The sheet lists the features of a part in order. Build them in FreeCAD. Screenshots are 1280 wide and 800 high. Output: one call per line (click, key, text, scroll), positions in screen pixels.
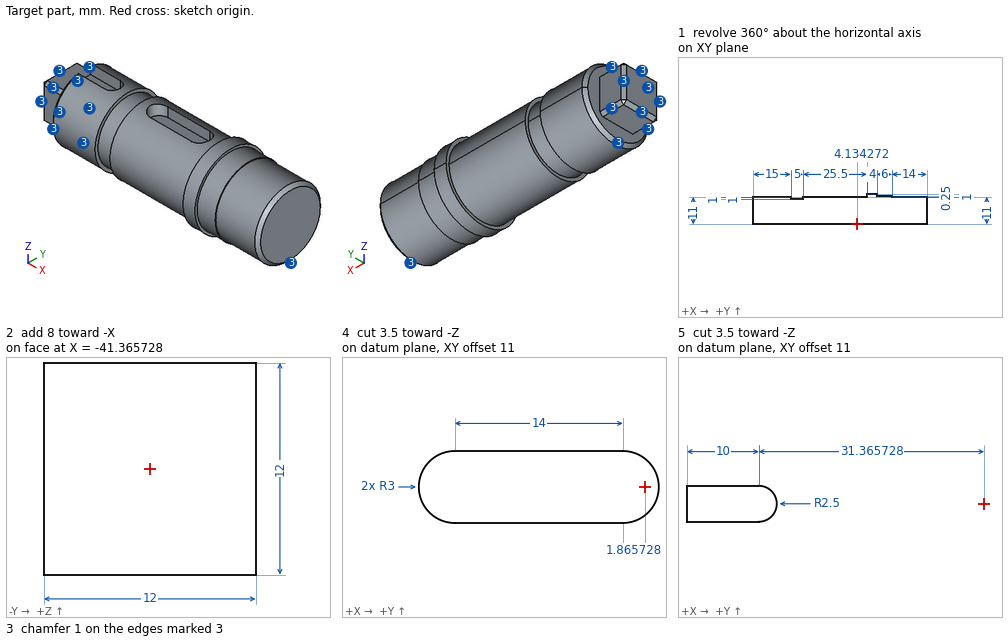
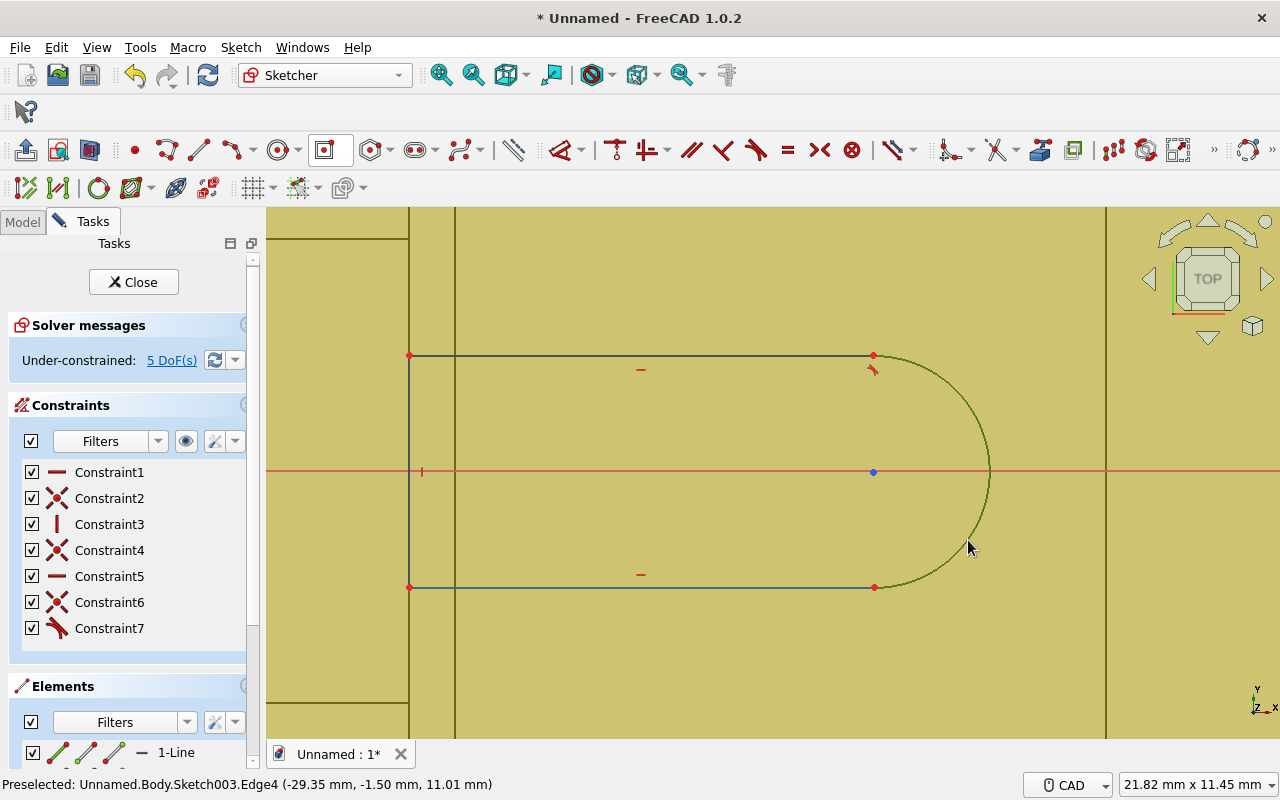
click(756, 150)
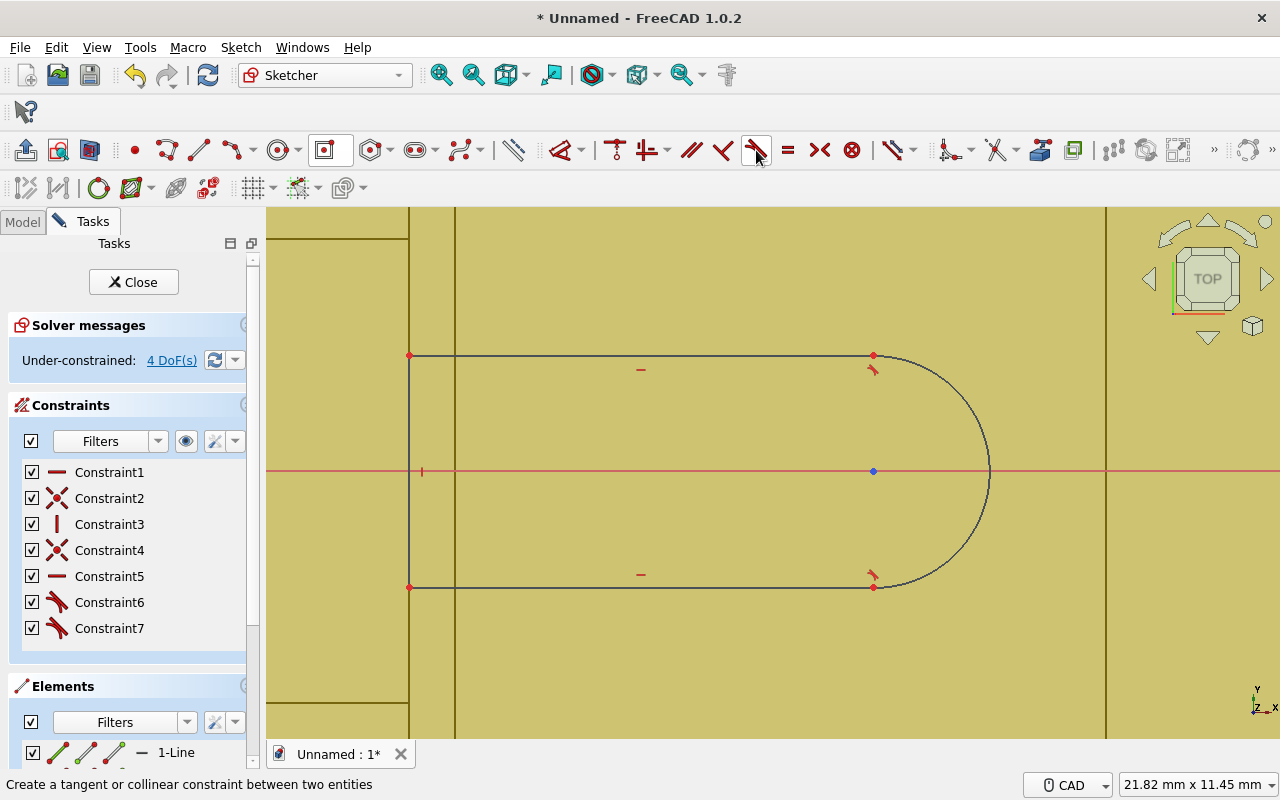
click(874, 472)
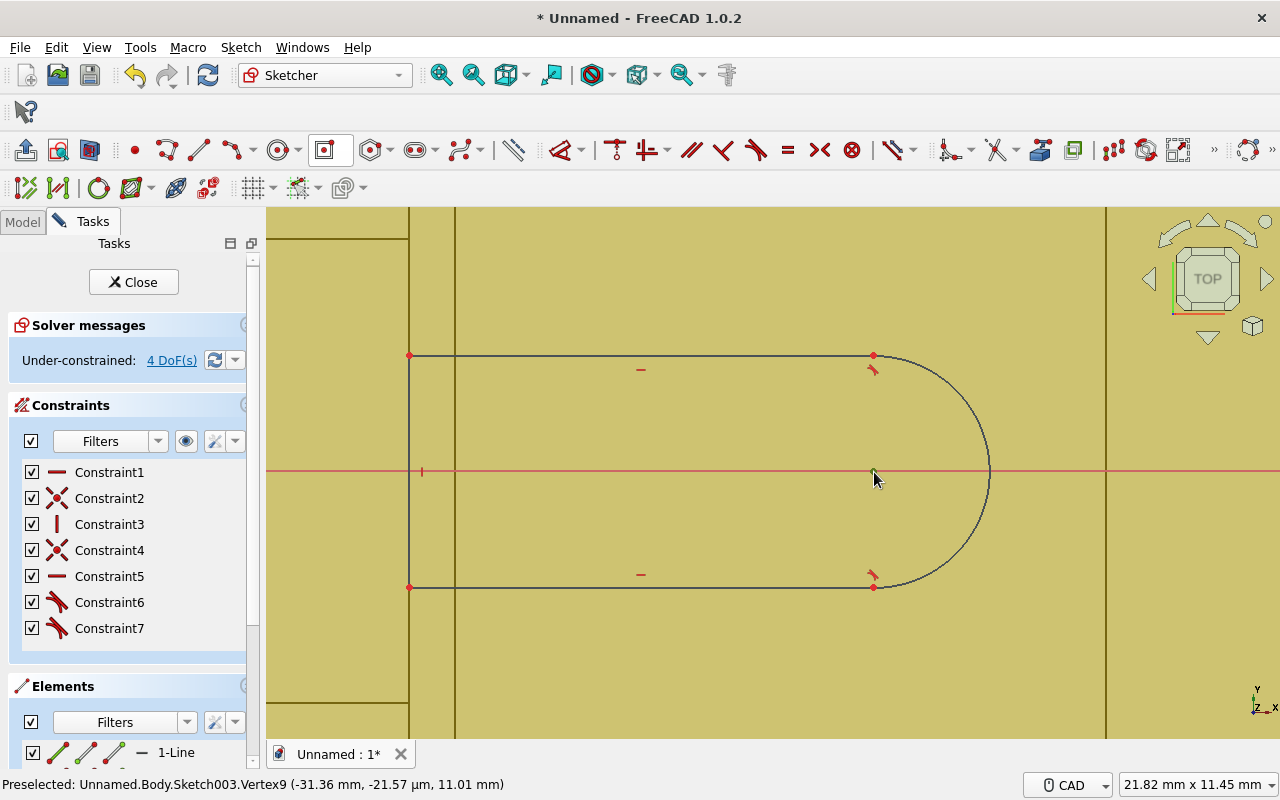
click(353, 471)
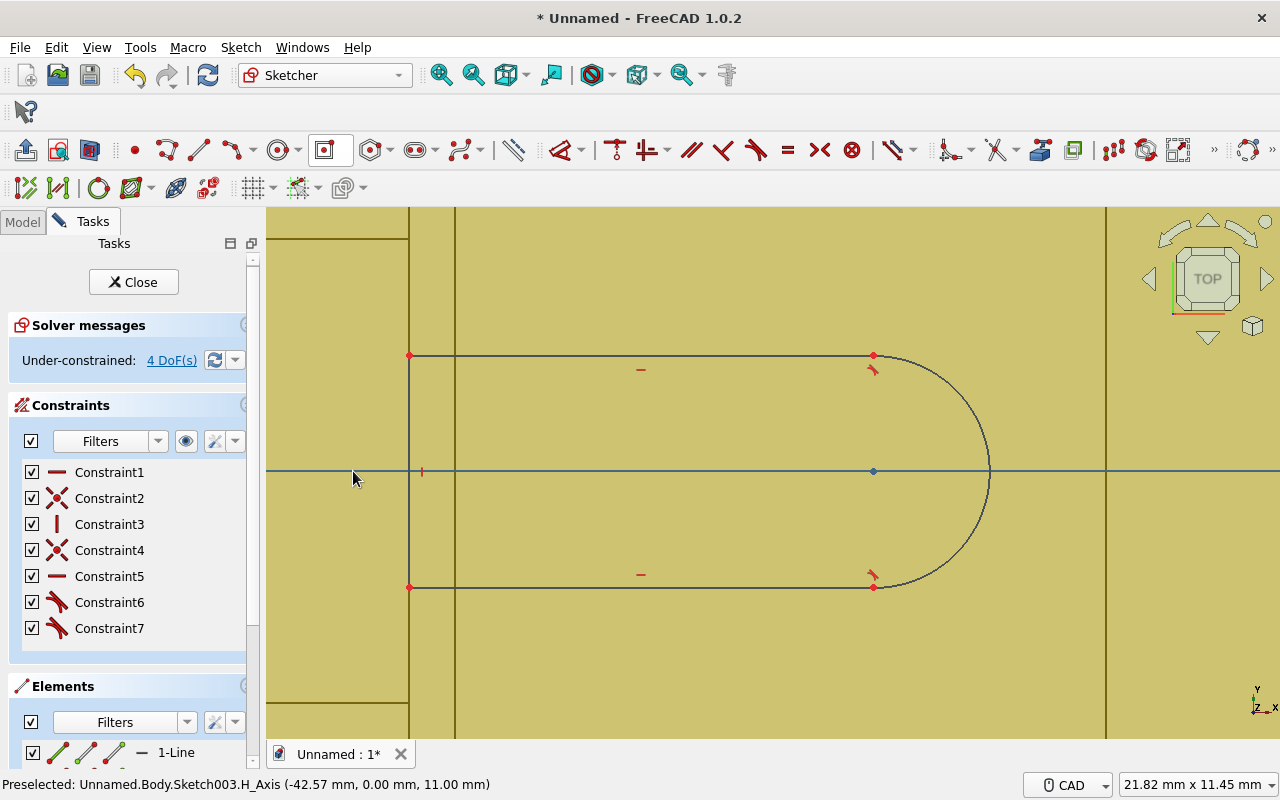
click(616, 150)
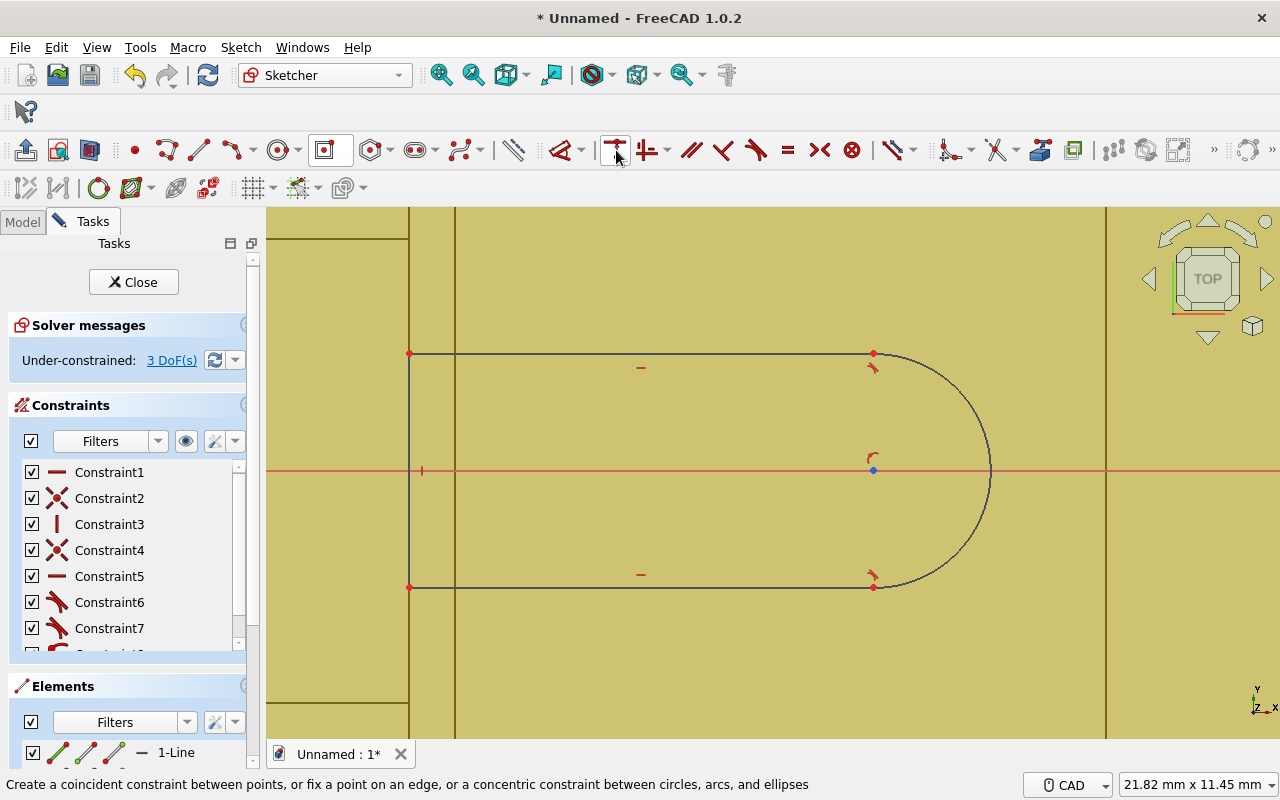
click(560, 150)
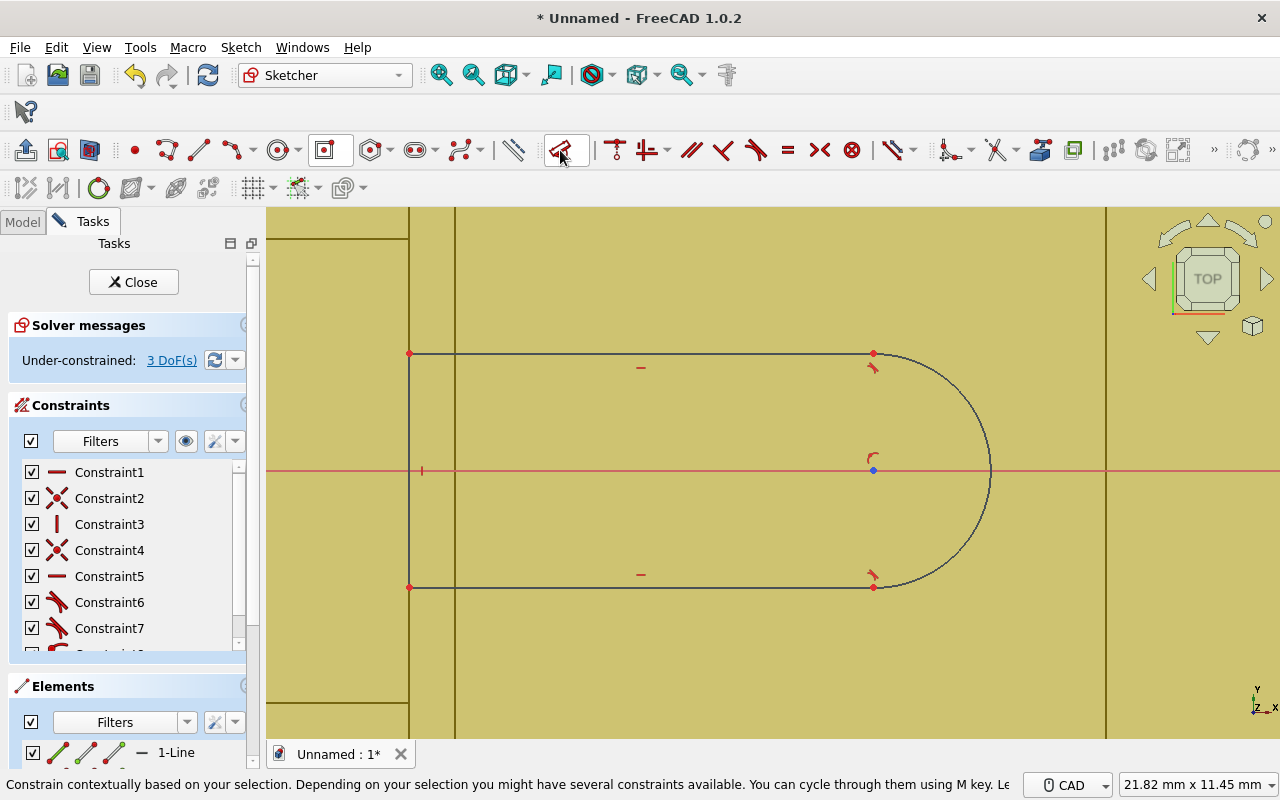
click(968, 540)
click(994, 559)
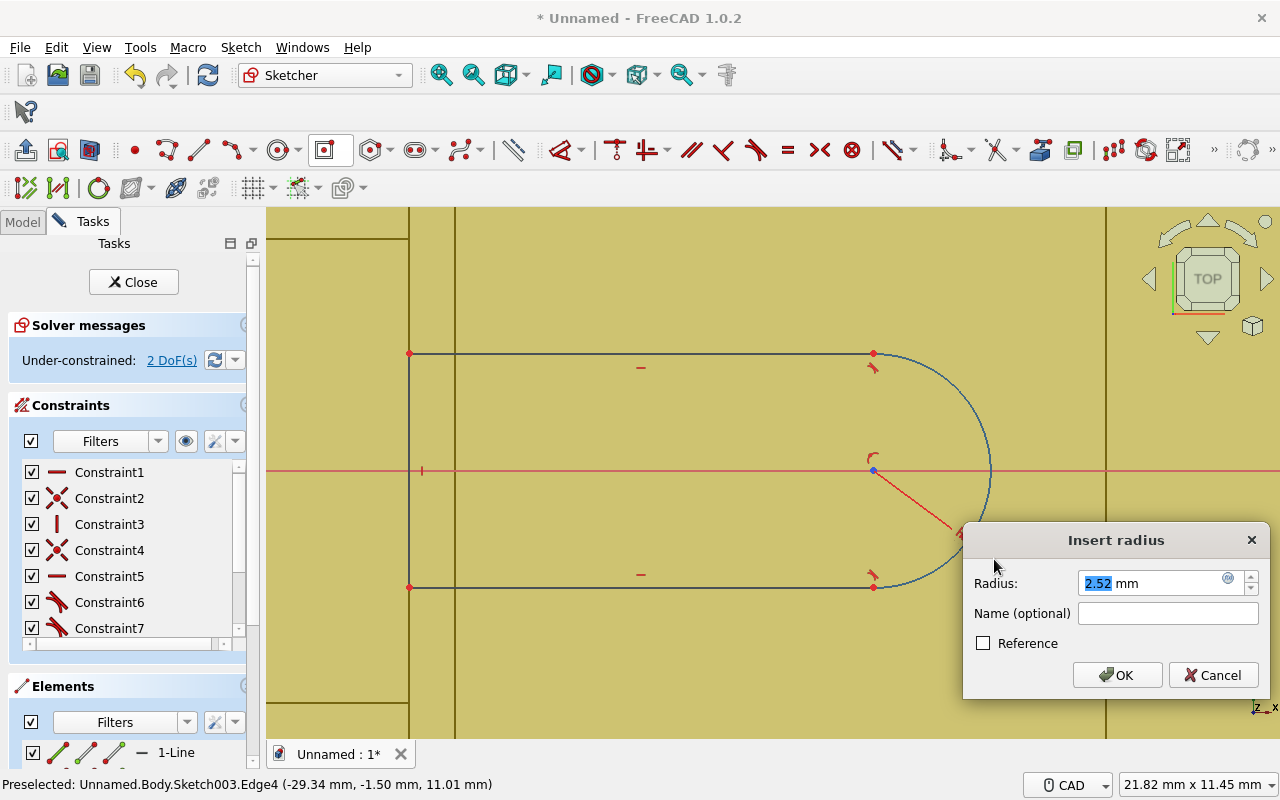
text(2.5)
key(Return)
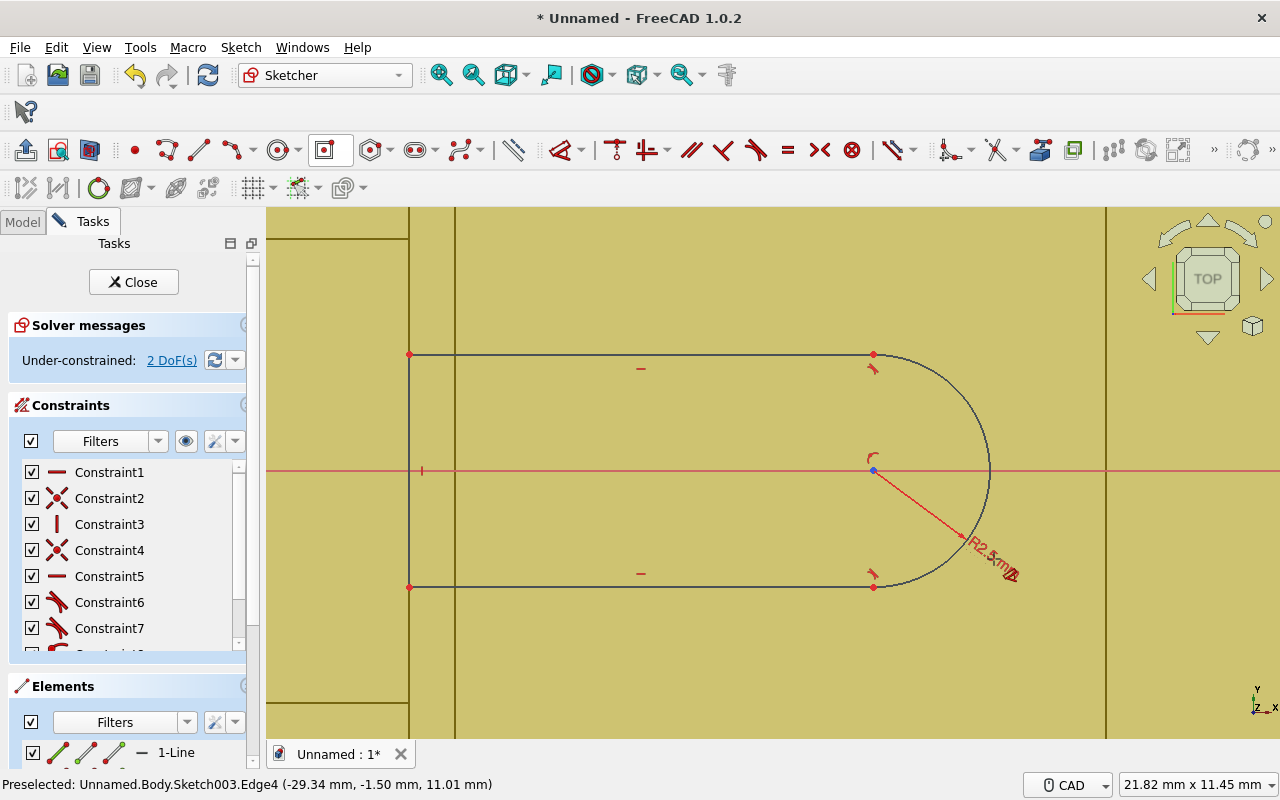
click(734, 355)
click(641, 321)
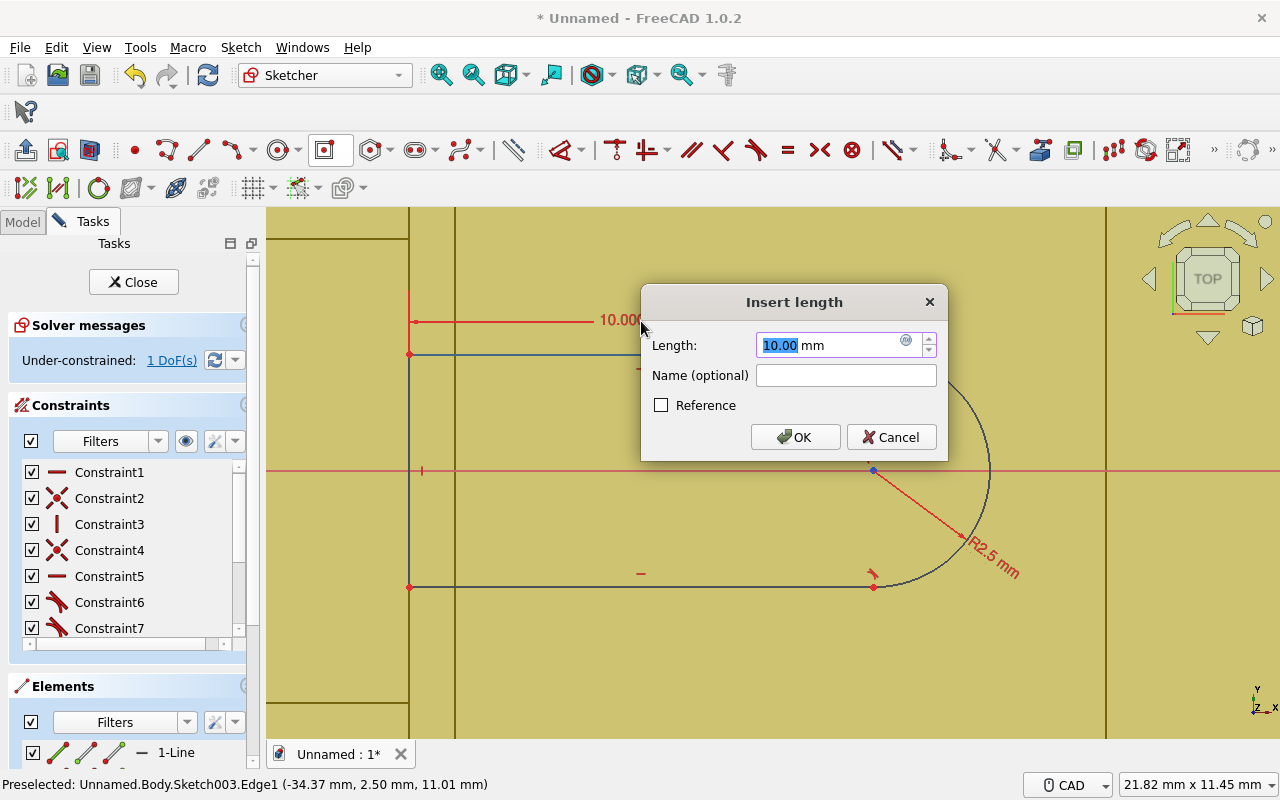
text(10)
key(Return)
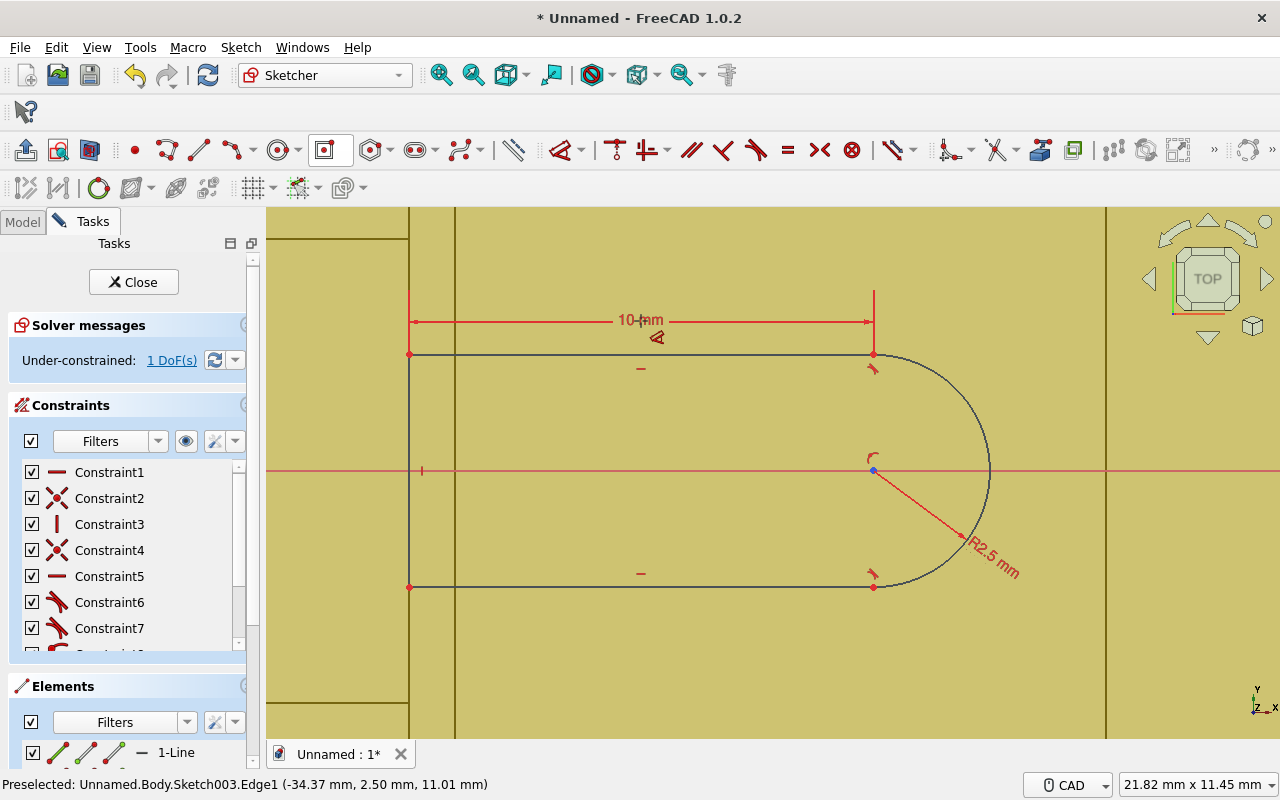
click(874, 355)
click(994, 321)